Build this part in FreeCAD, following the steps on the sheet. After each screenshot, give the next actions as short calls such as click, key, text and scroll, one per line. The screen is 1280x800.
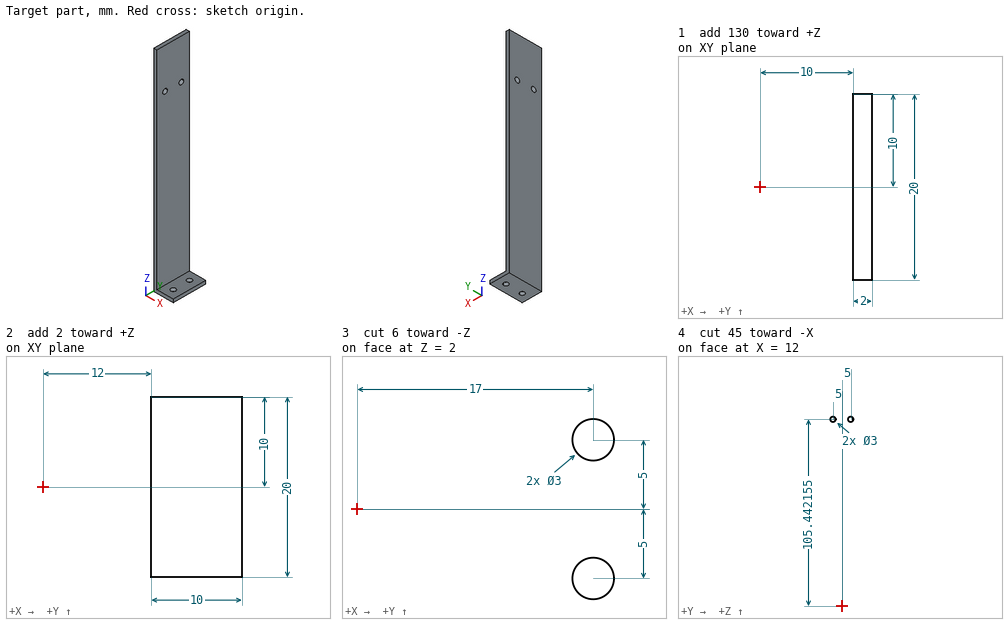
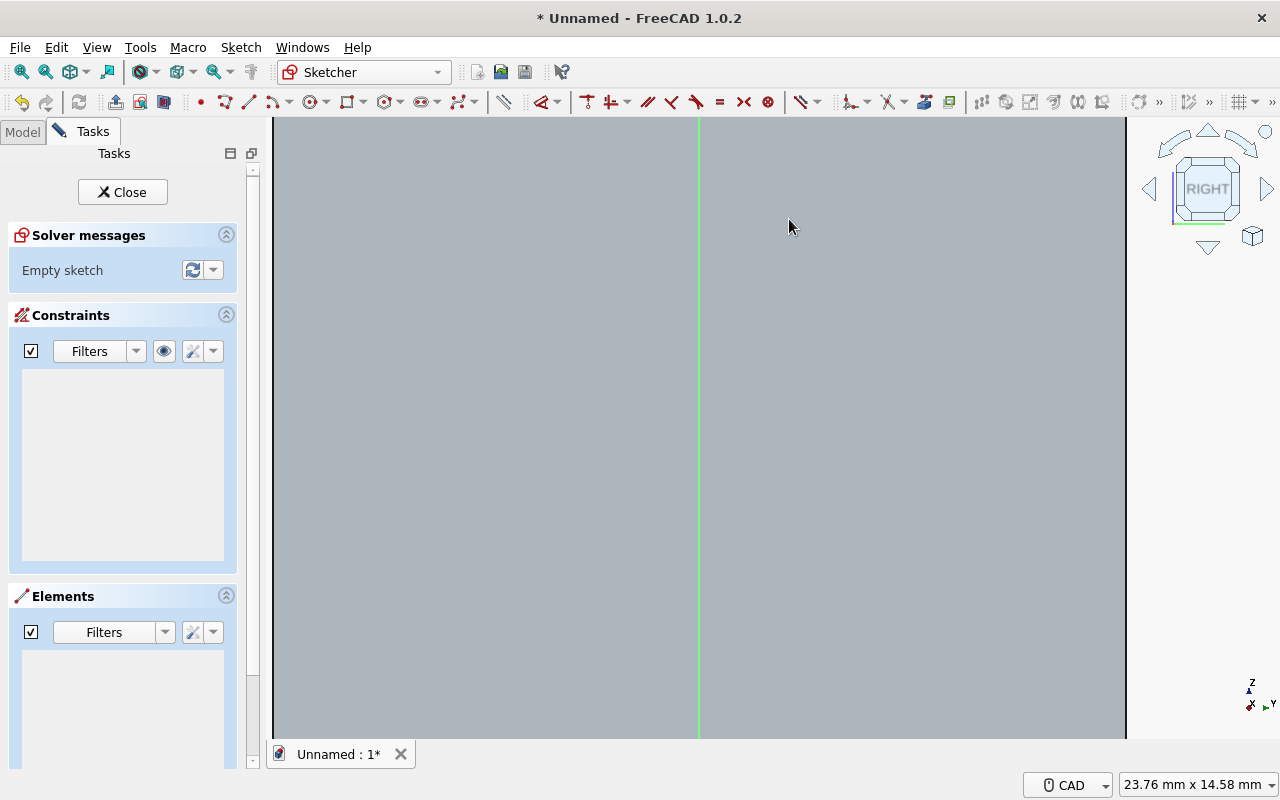
click(310, 102)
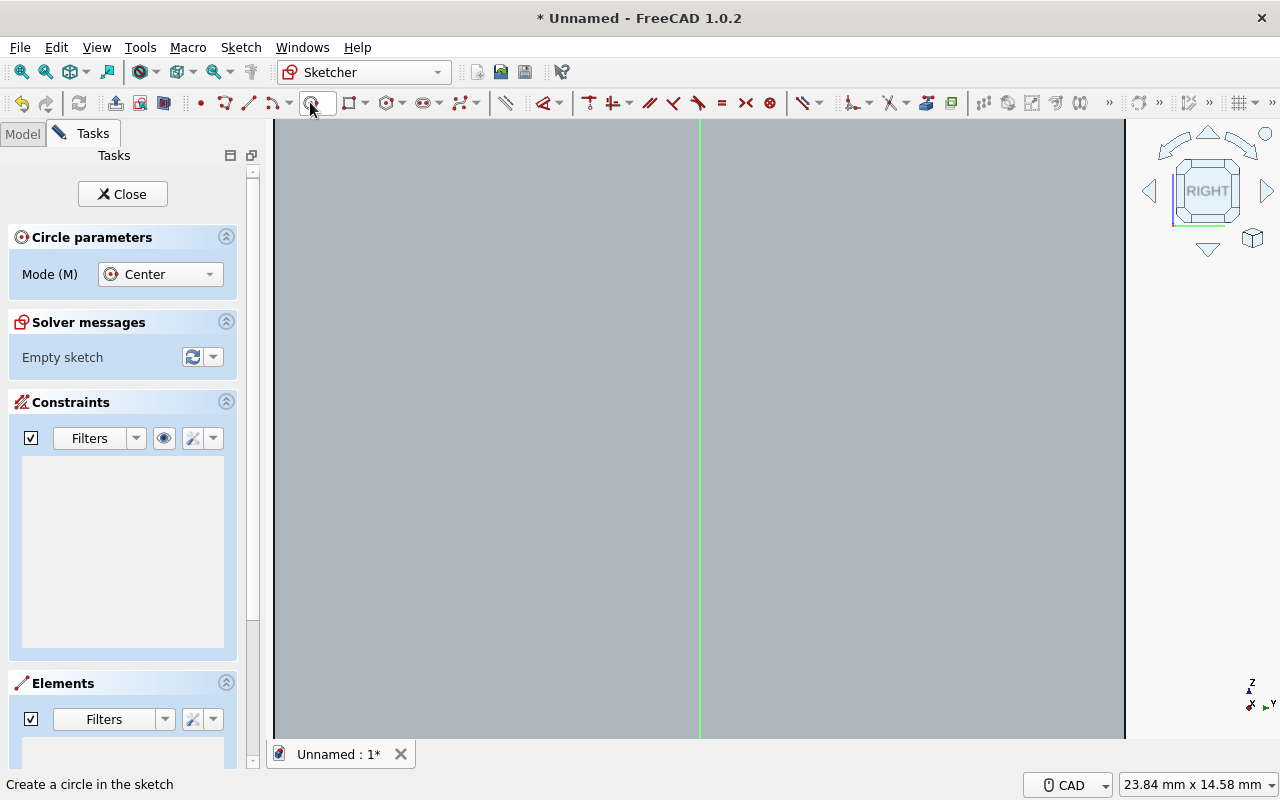
click(487, 427)
move(532, 382)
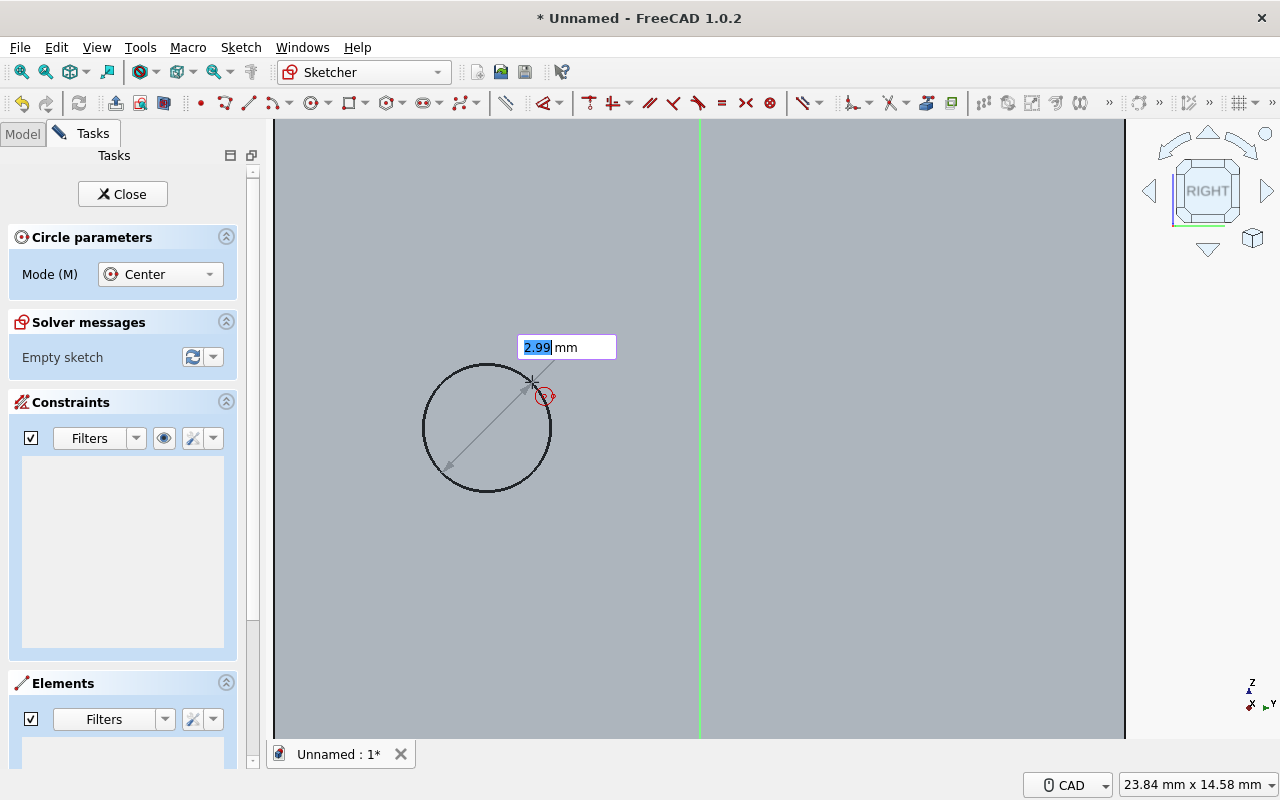
text(3)
key(Return)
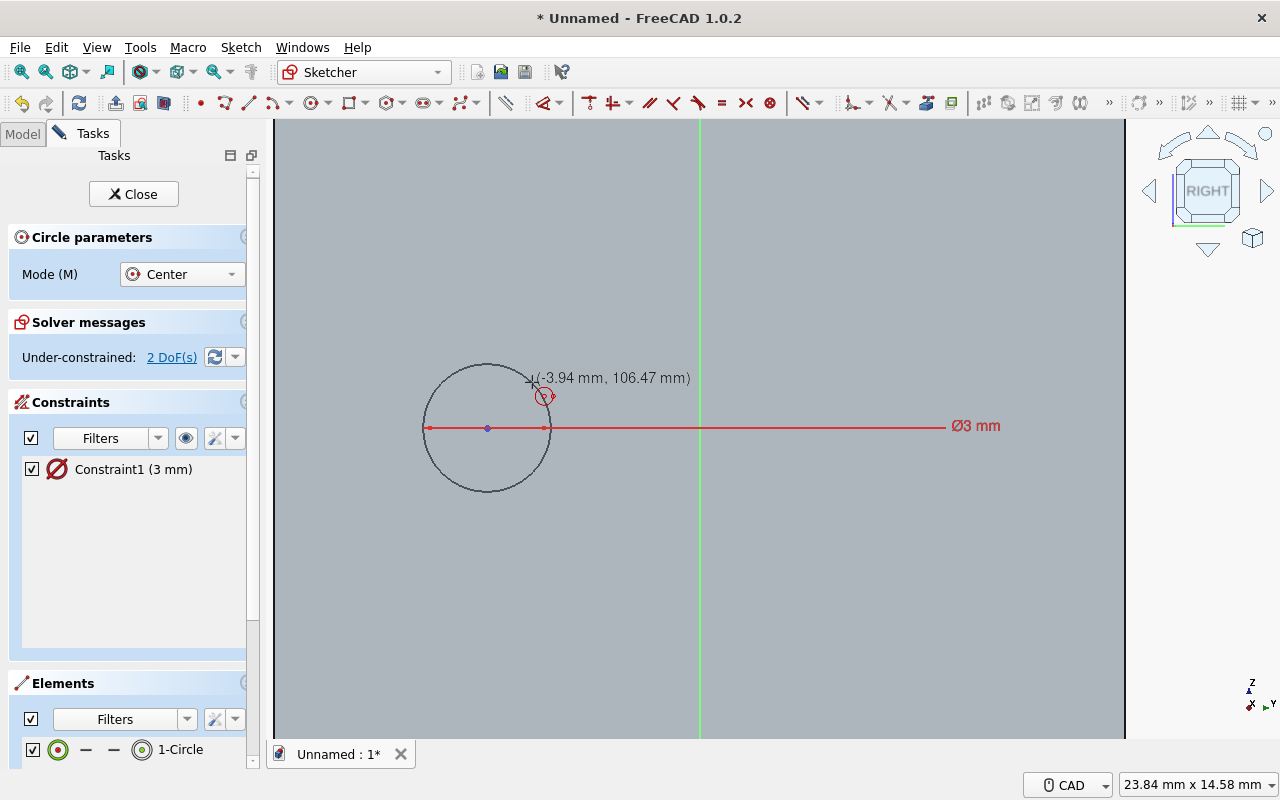
click(912, 427)
move(957, 382)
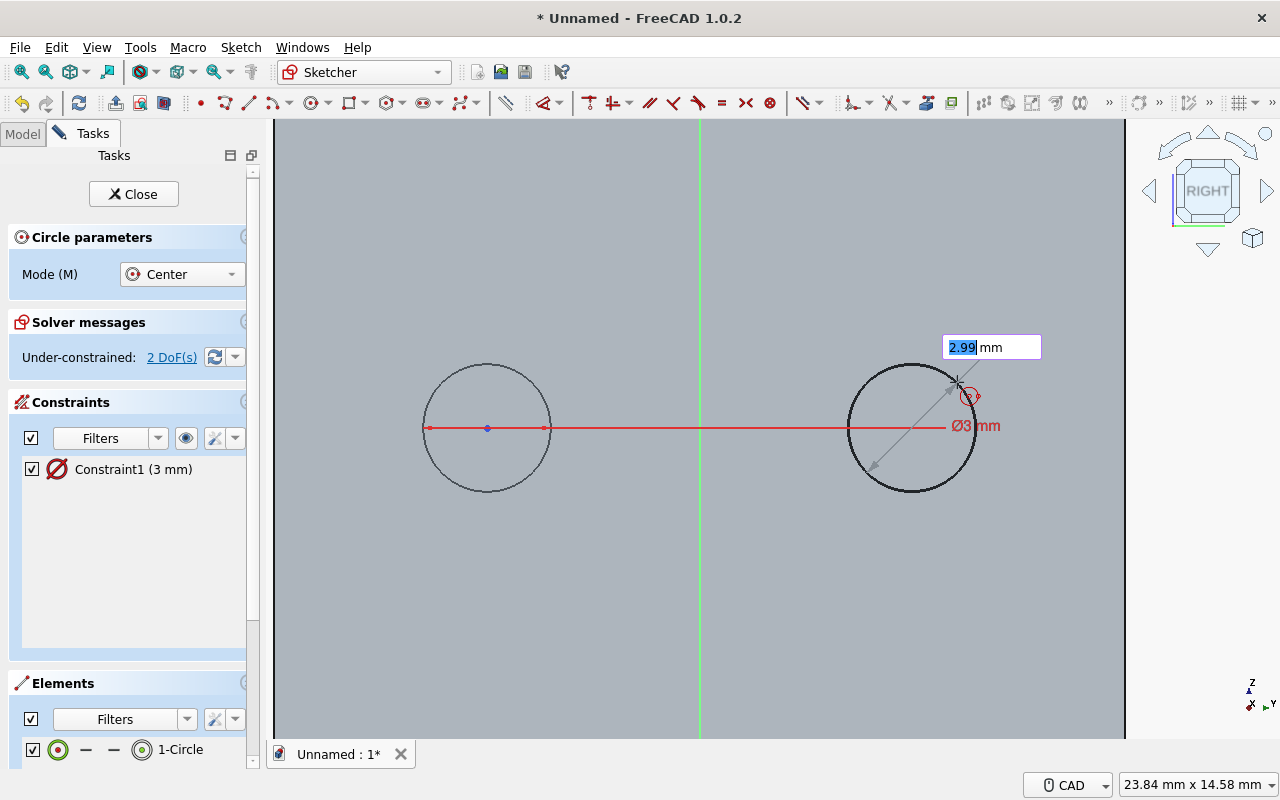
text(3)
key(Return)
key(Escape)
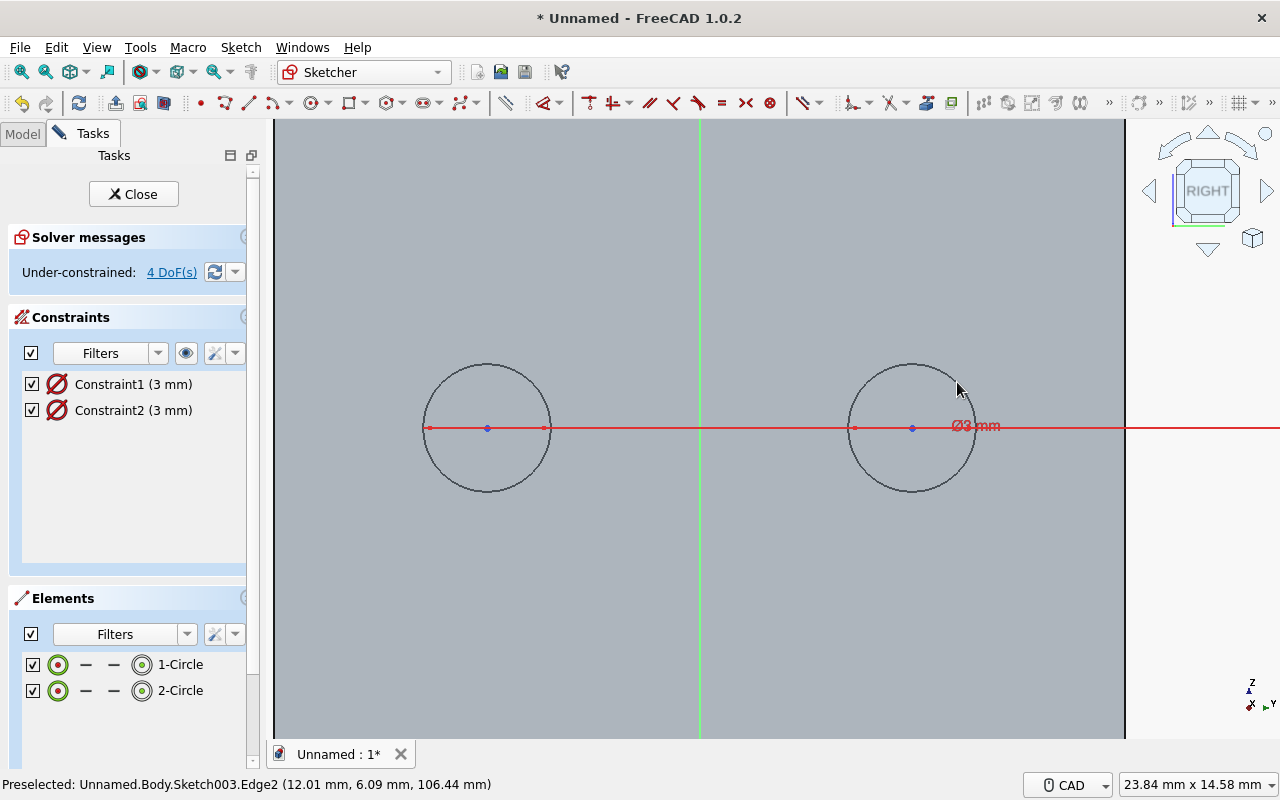
click(487, 428)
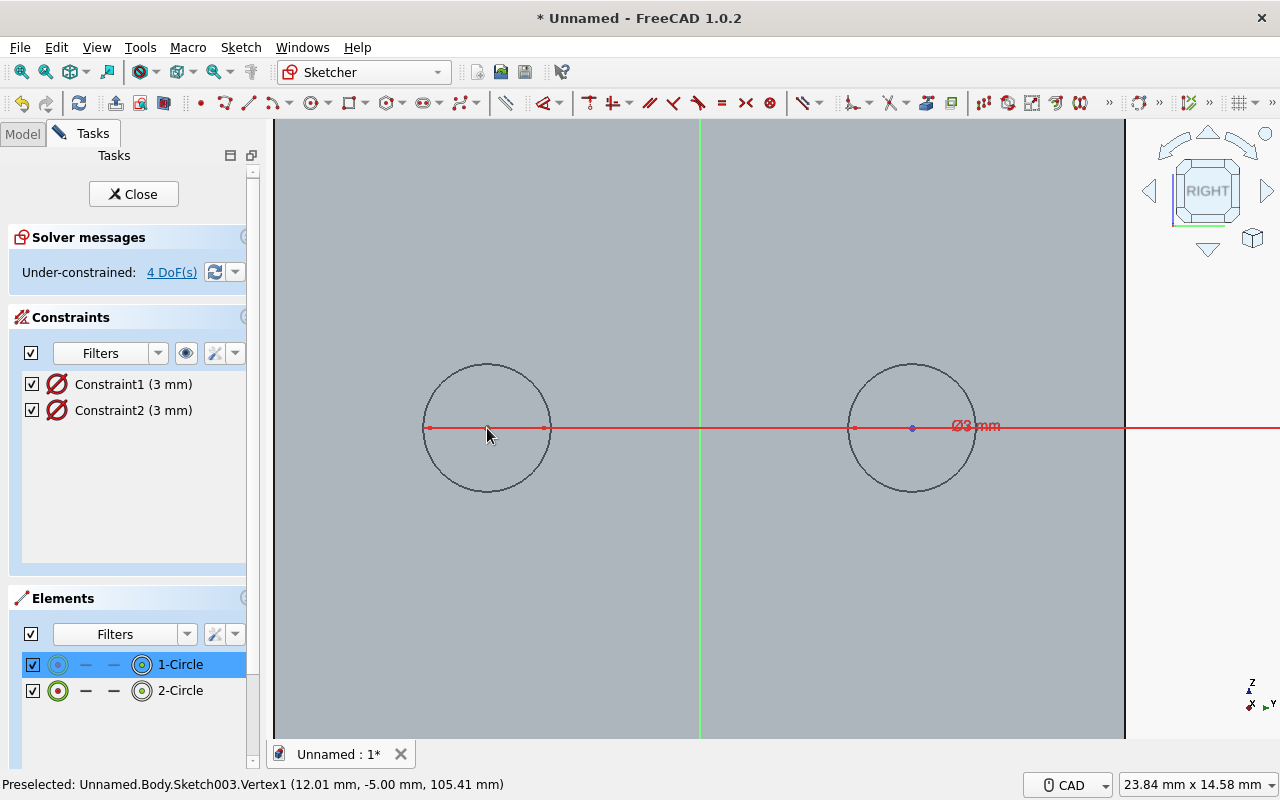
click(912, 428)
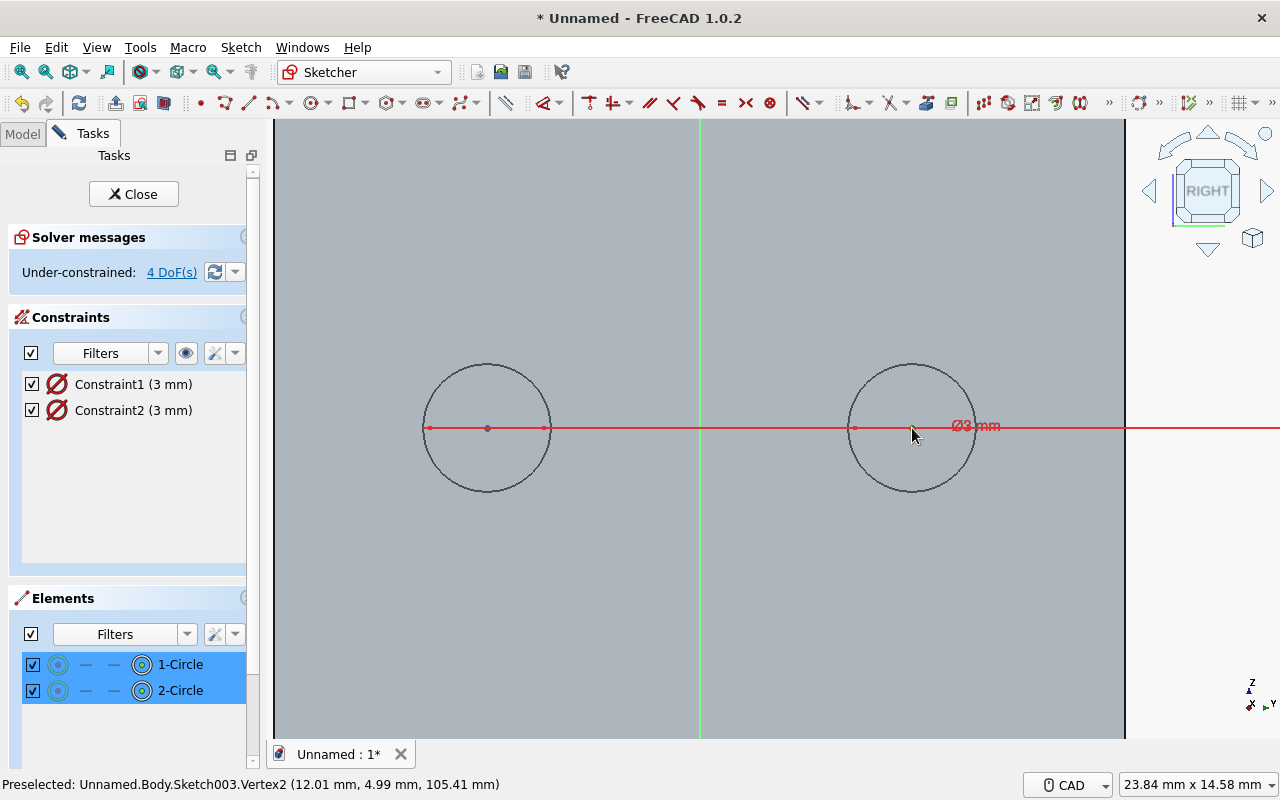
key(h)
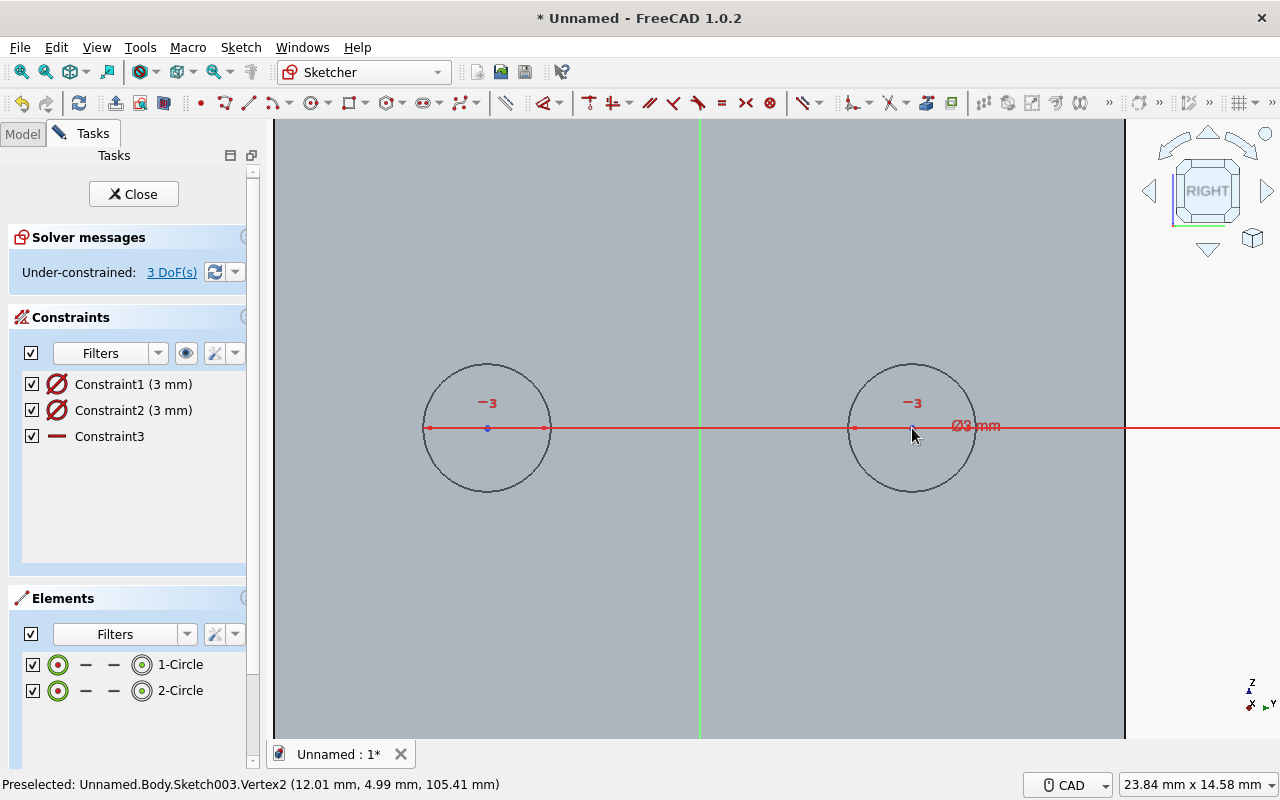
click(544, 104)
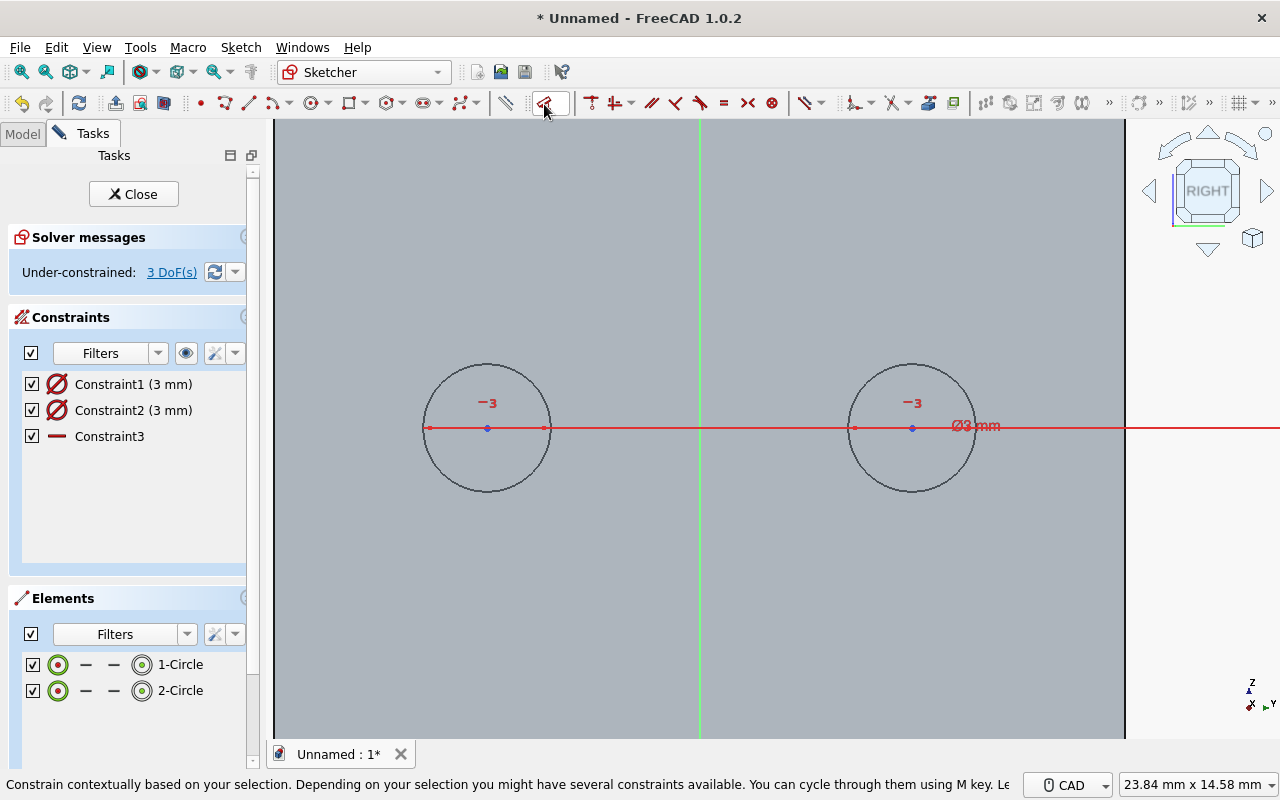
click(487, 428)
click(593, 394)